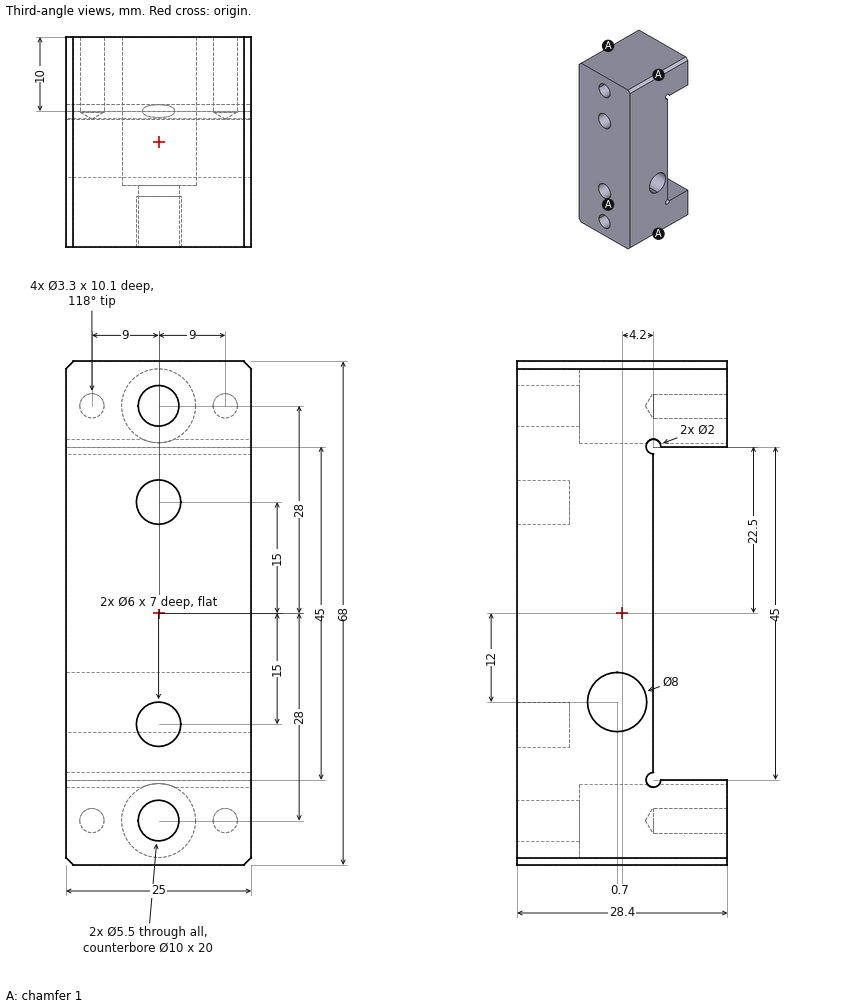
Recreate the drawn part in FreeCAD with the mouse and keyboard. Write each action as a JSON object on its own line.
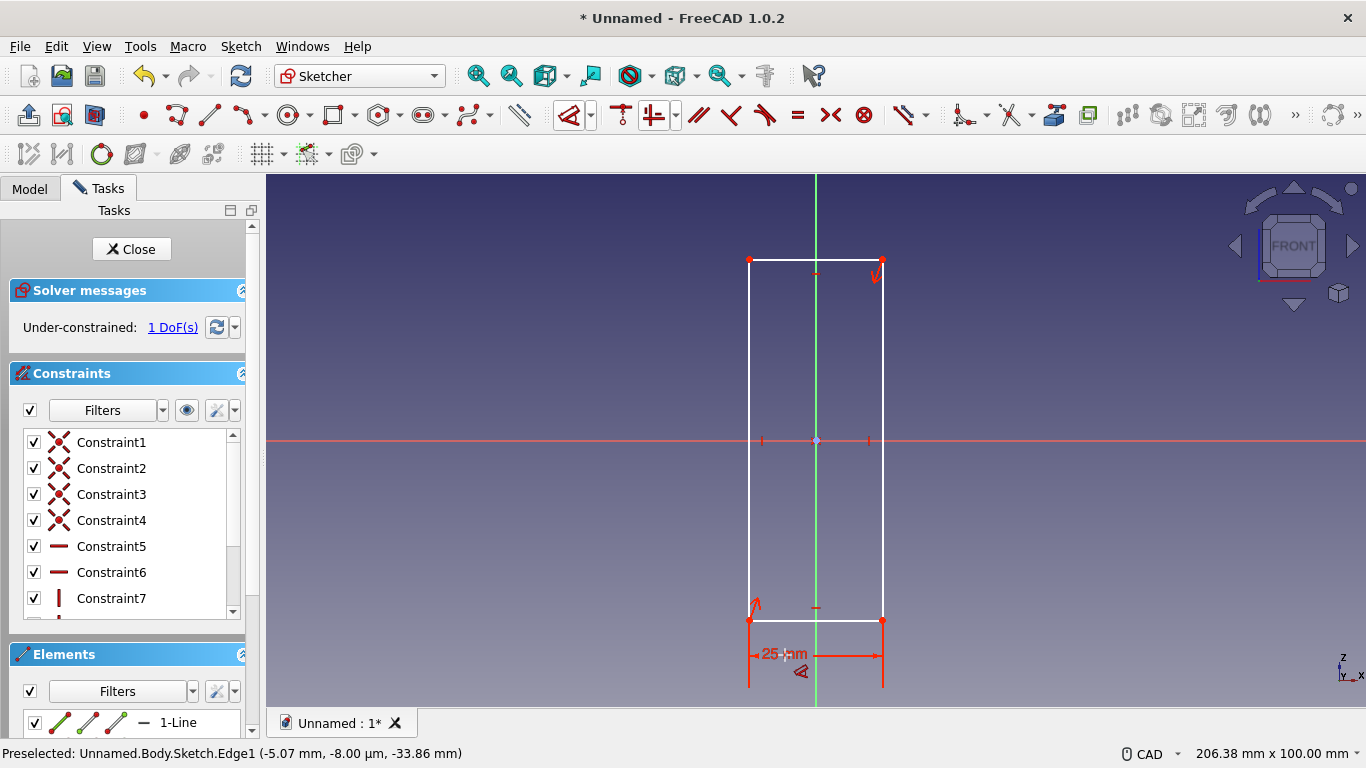
{"action": "left_click", "coordinate": [883, 513]}
{"action": "left_click", "coordinate": [917, 357]}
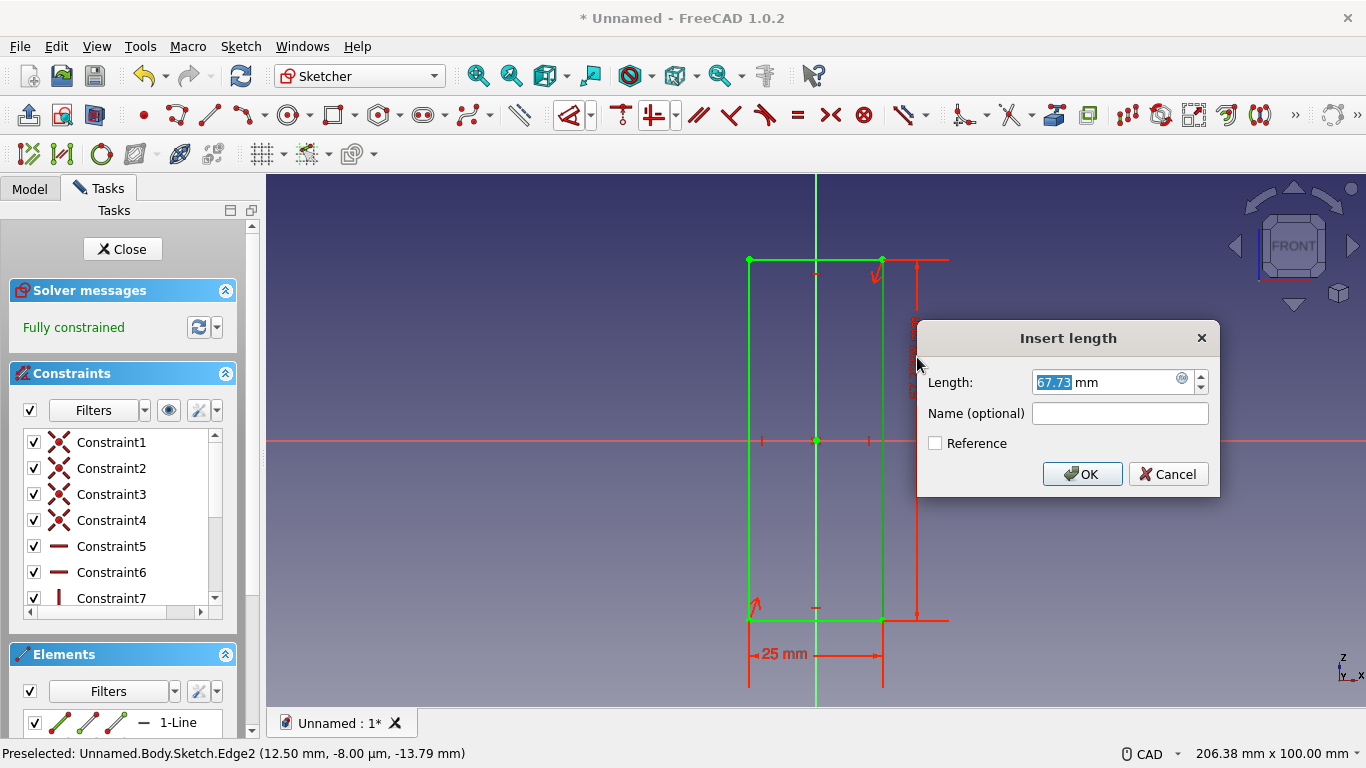
{"action": "type", "text": "68"}
{"action": "key", "text": "Return"}
{"action": "key", "text": "Escape"}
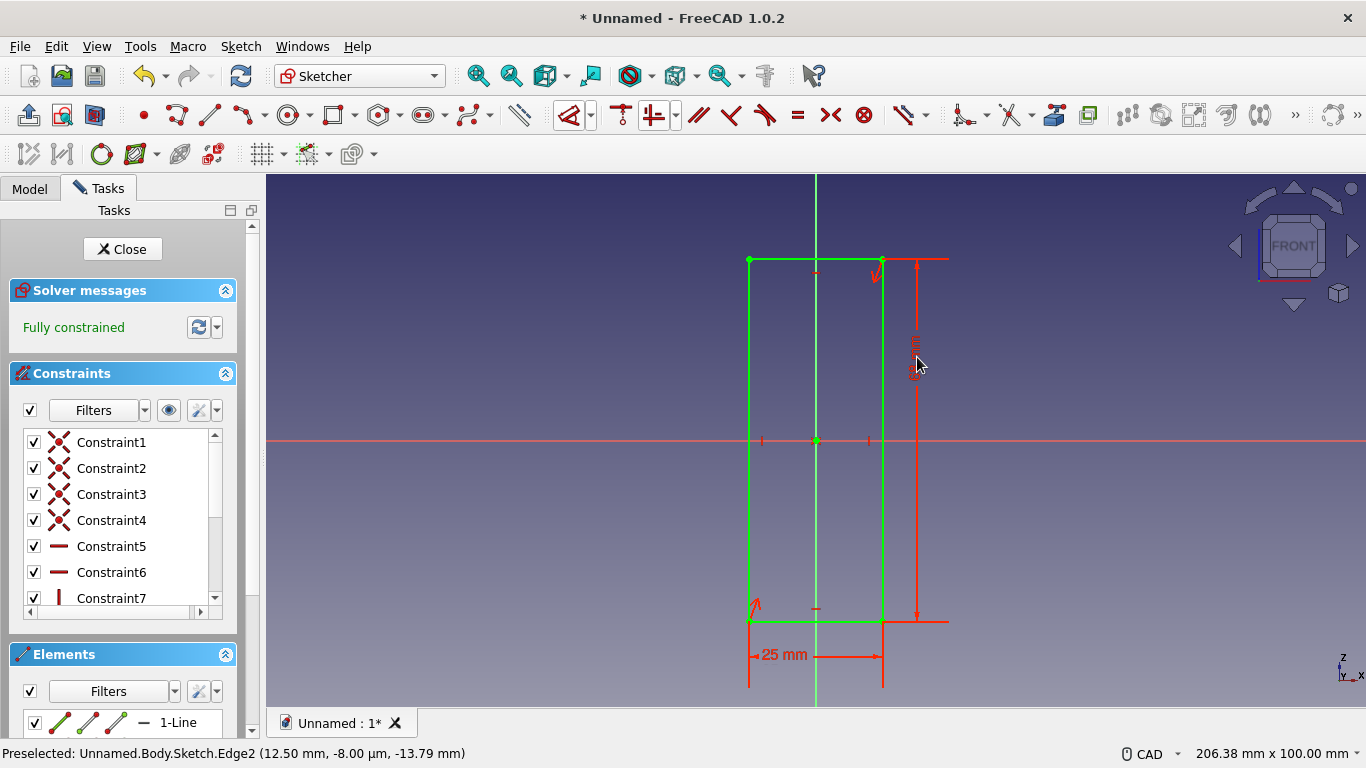
{"action": "left_click", "coordinate": [123, 249]}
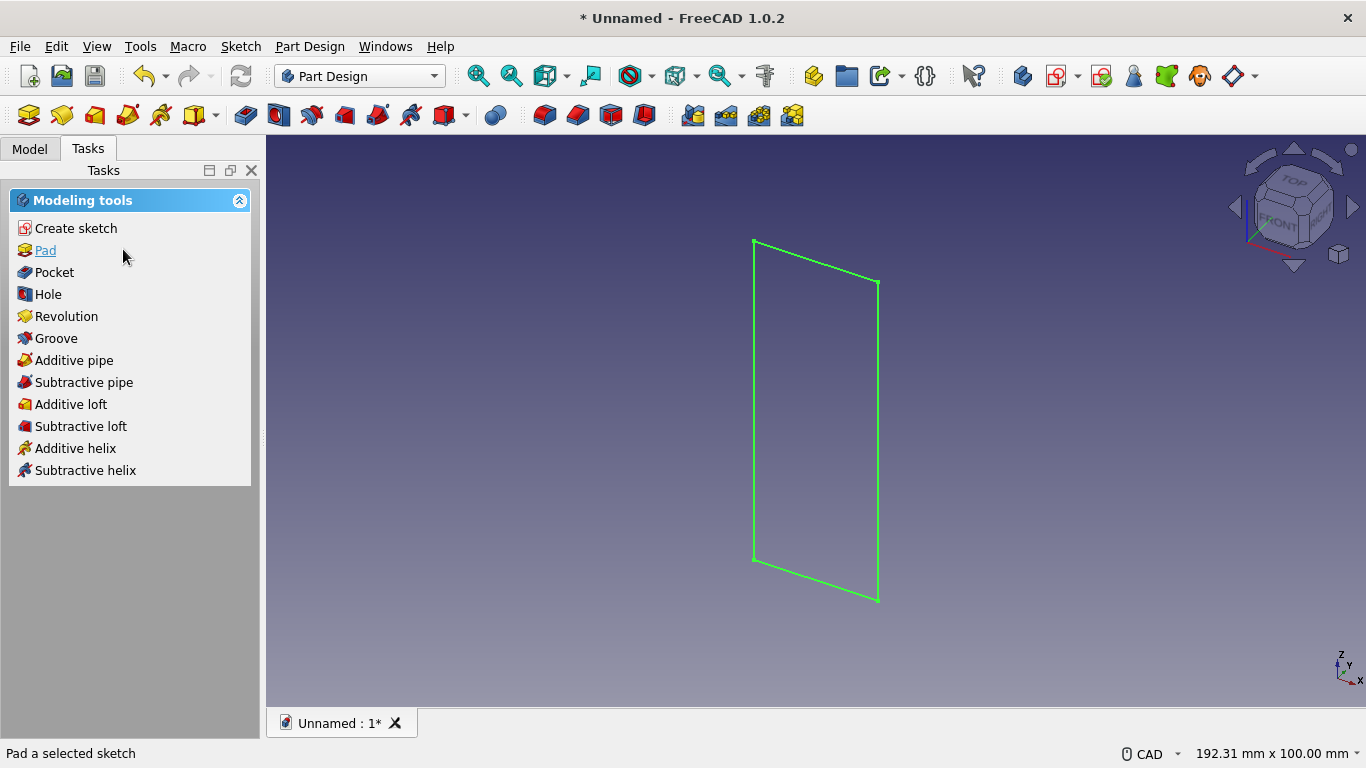
{"action": "left_click", "coordinate": [29, 116]}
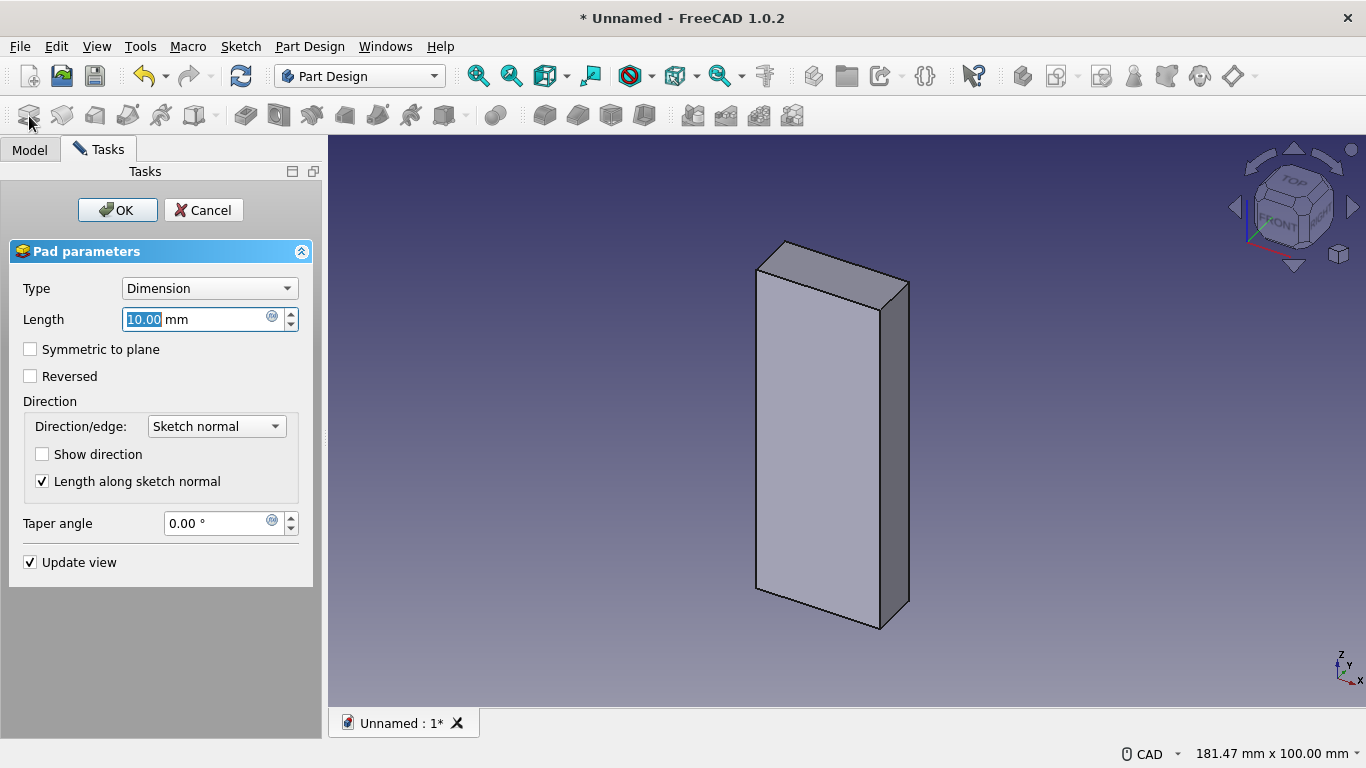
{"action": "type", "text": "28.4"}
{"action": "key", "text": "Tab"}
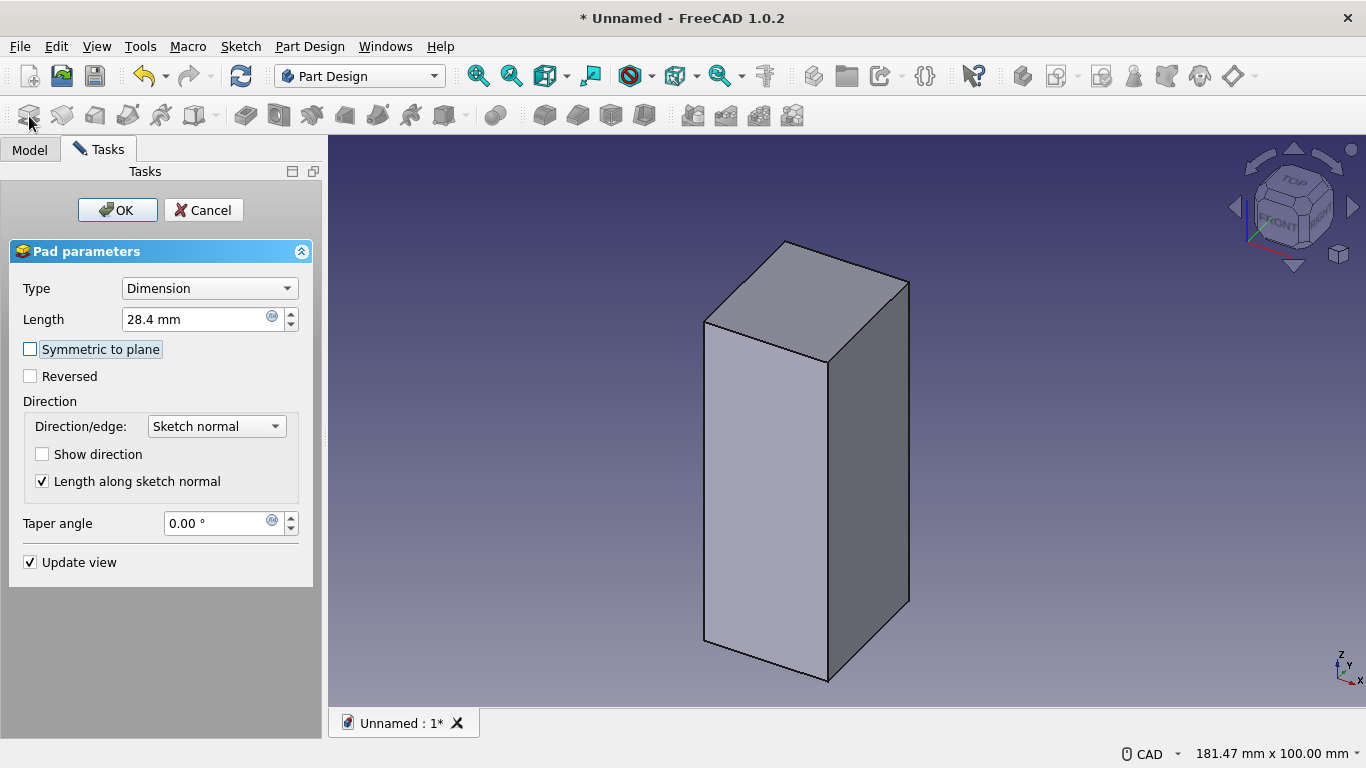
{"action": "left_click", "coordinate": [31, 349]}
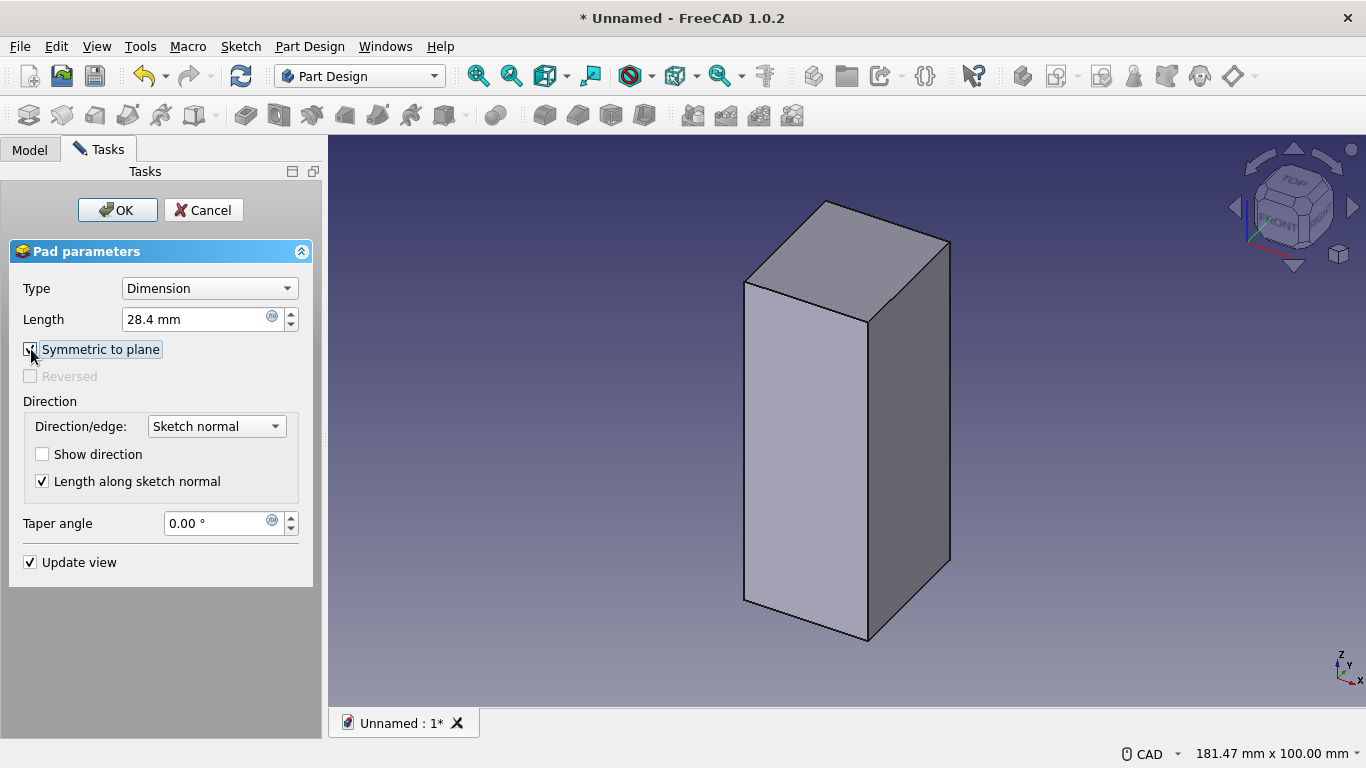
{"action": "left_click", "coordinate": [118, 210]}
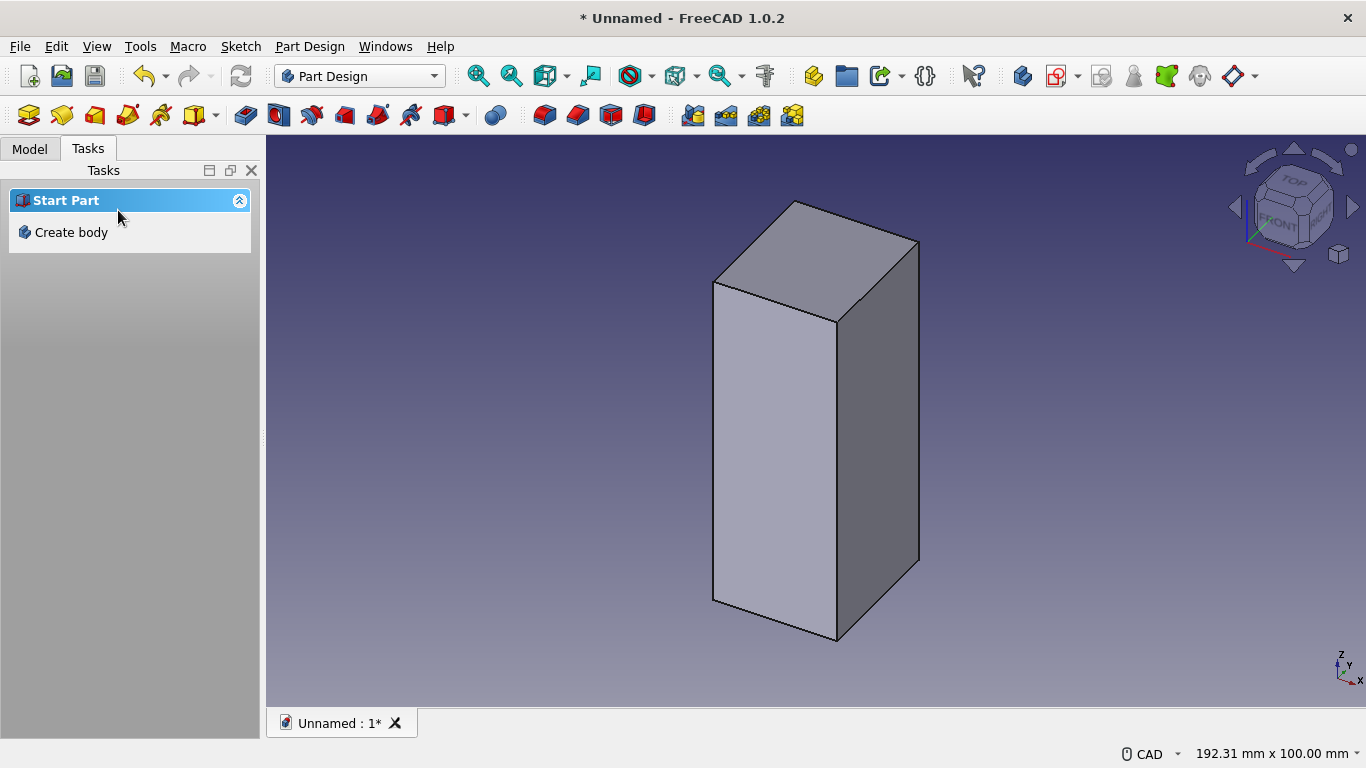
{"action": "key", "text": "4"}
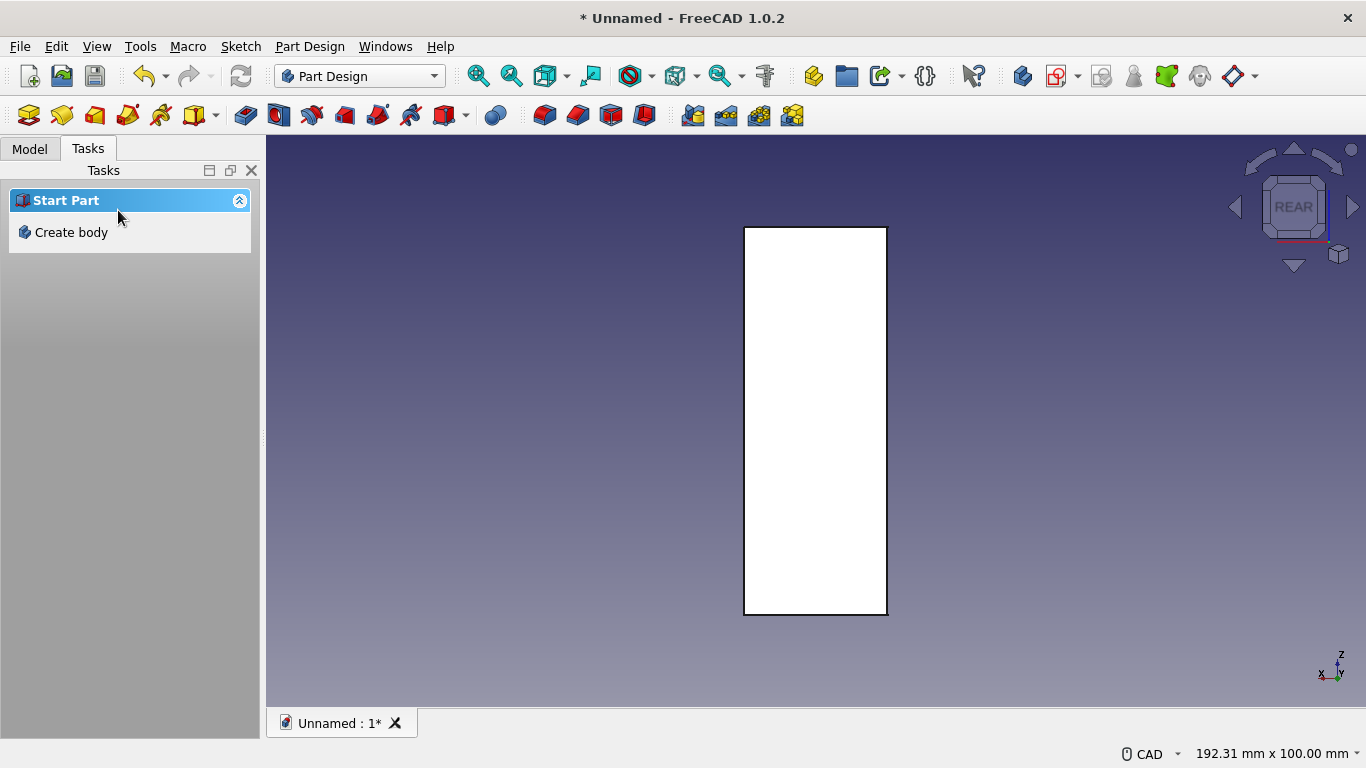
{"action": "left_click", "coordinate": [816, 309]}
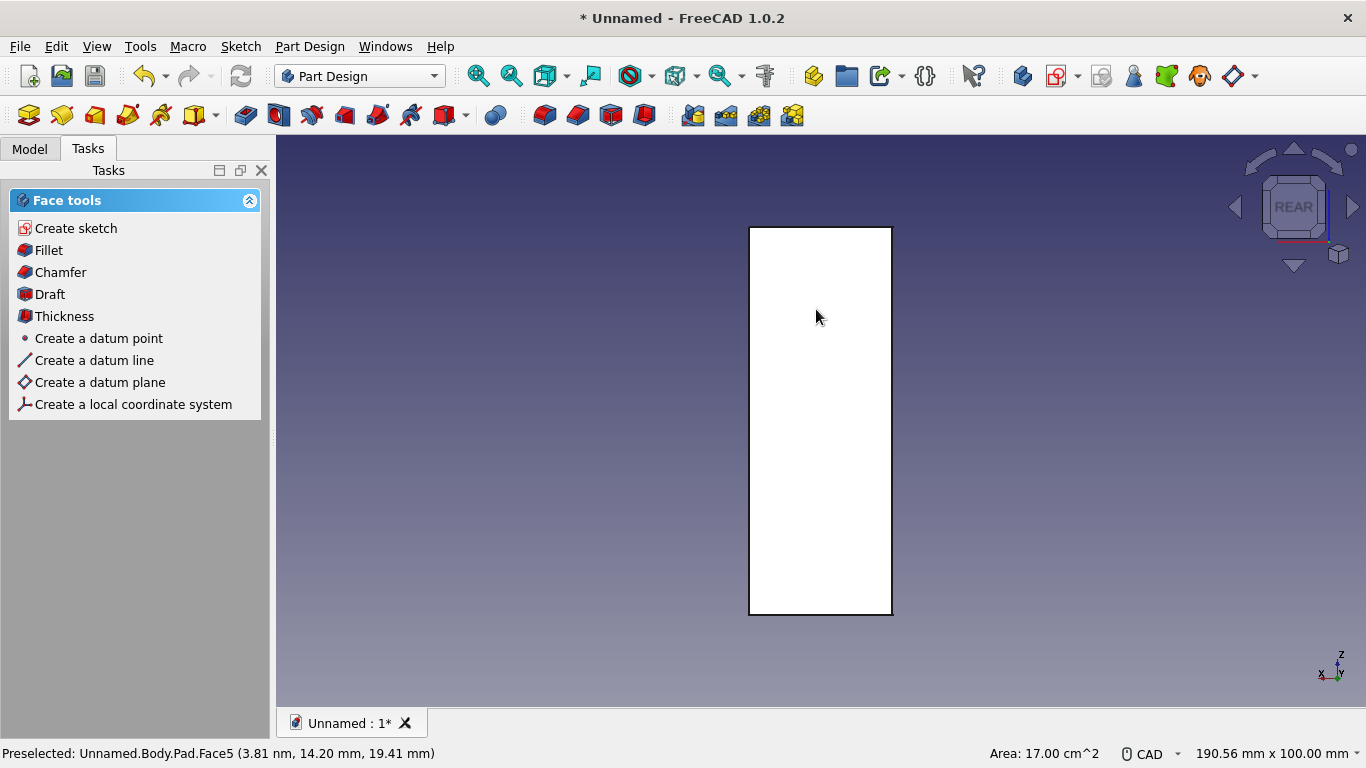
{"action": "left_click", "coordinate": [1056, 76]}